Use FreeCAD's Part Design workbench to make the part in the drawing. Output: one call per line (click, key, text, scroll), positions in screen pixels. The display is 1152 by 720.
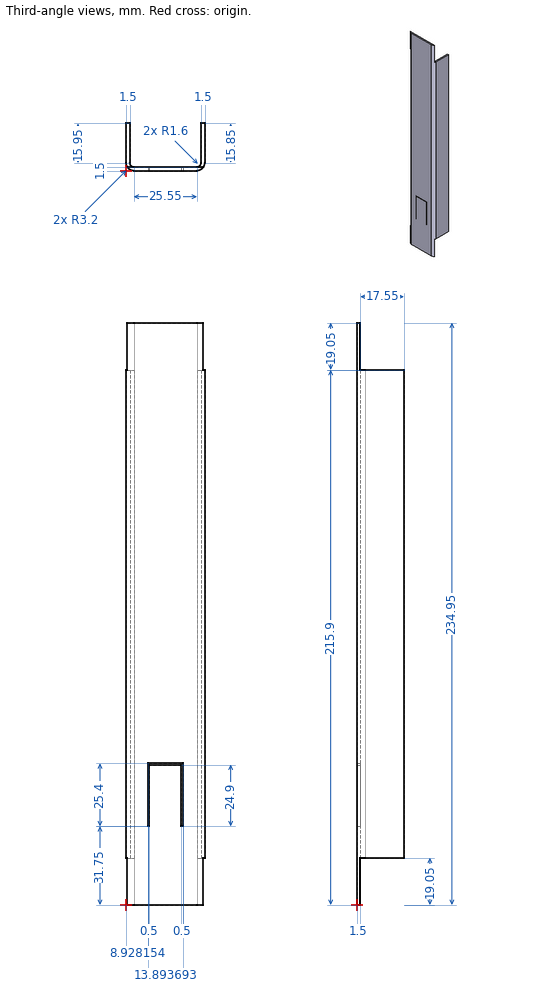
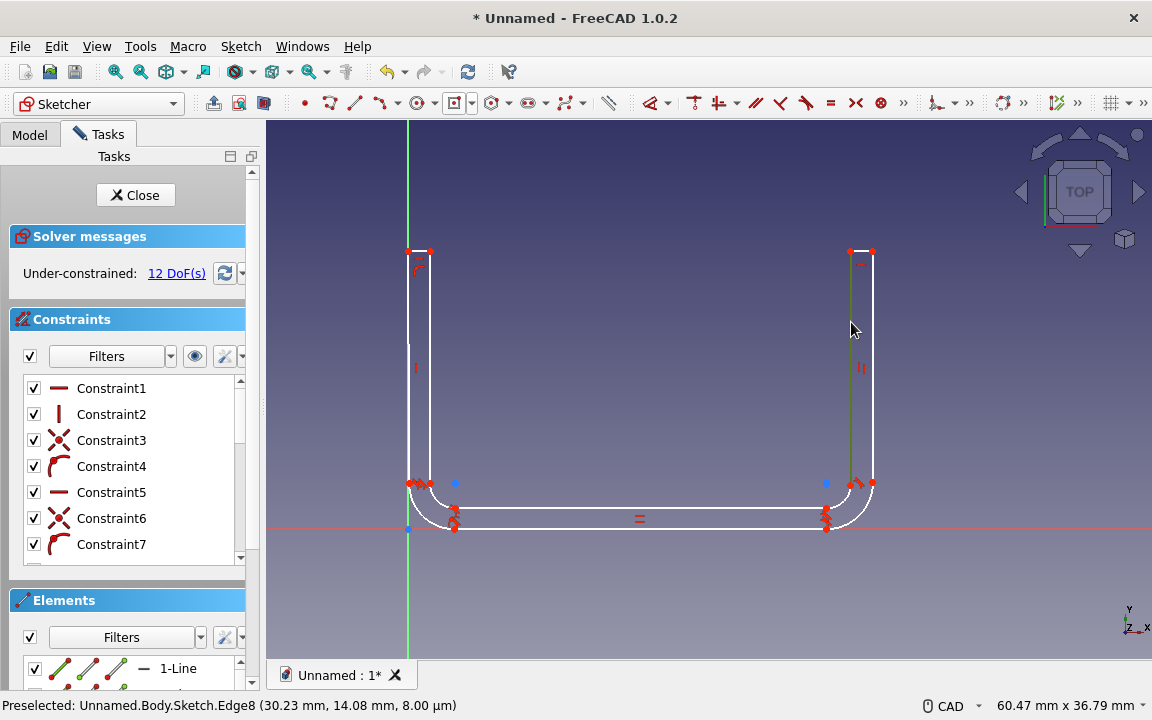
scroll(837, 506, up, 2)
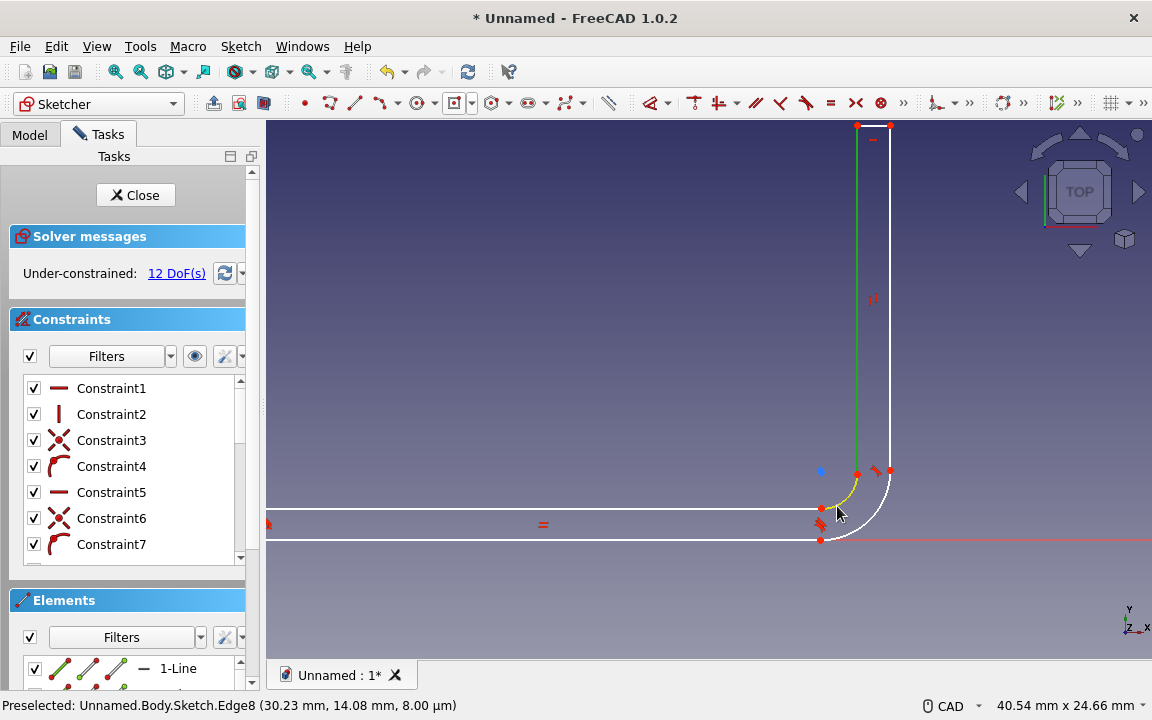
click(837, 505)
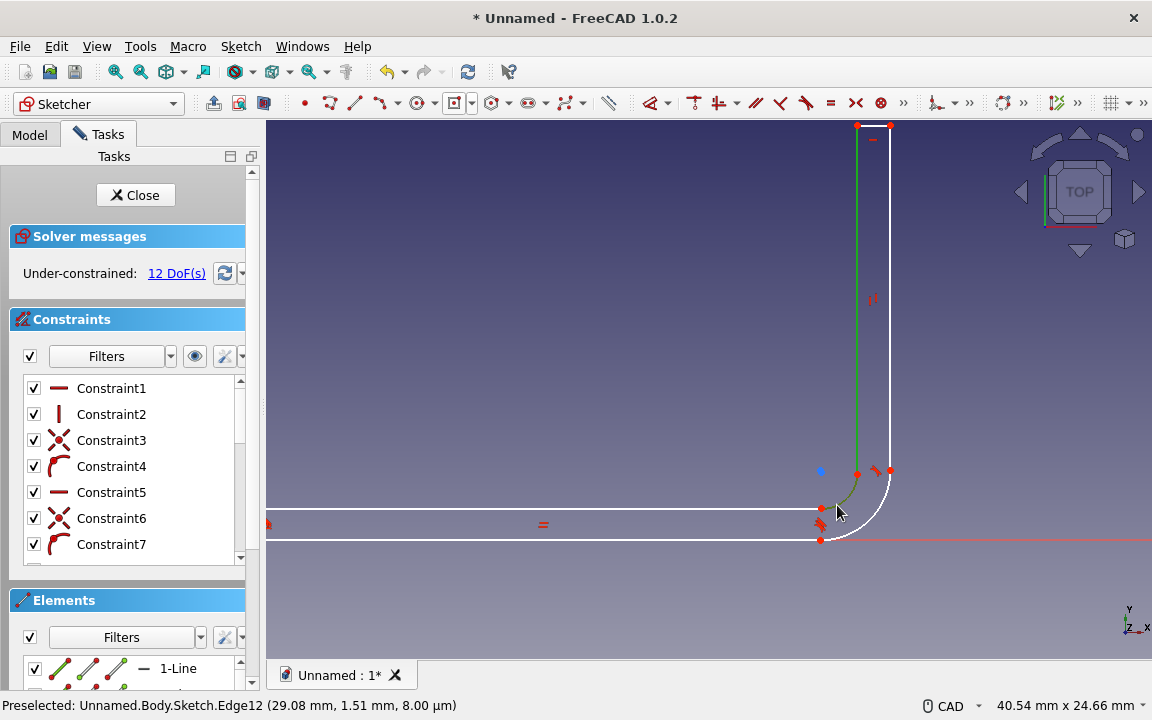
key(t)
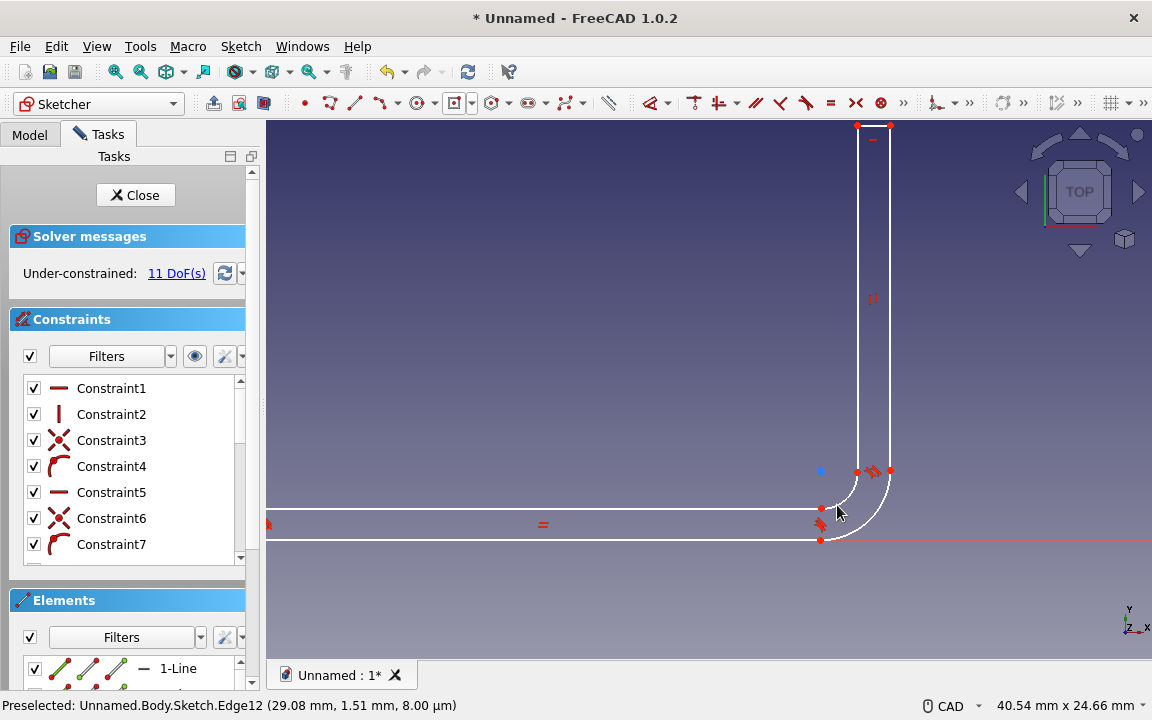
scroll(837, 506, down, 2)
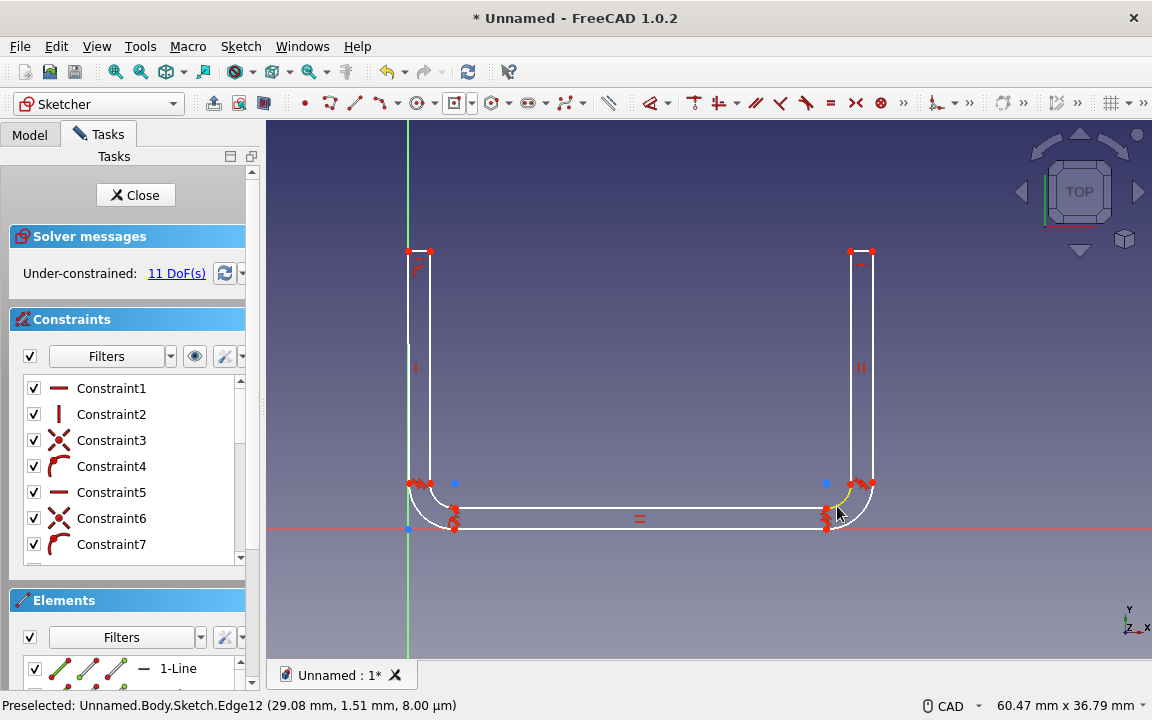
click(408, 321)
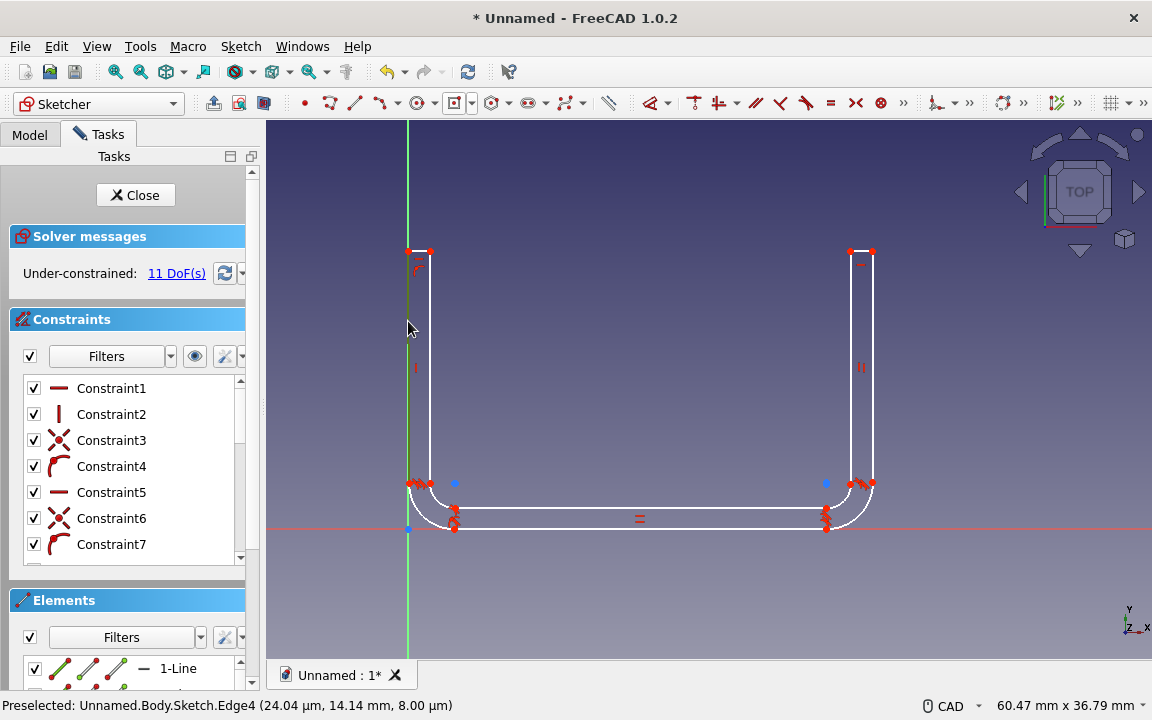
key(v)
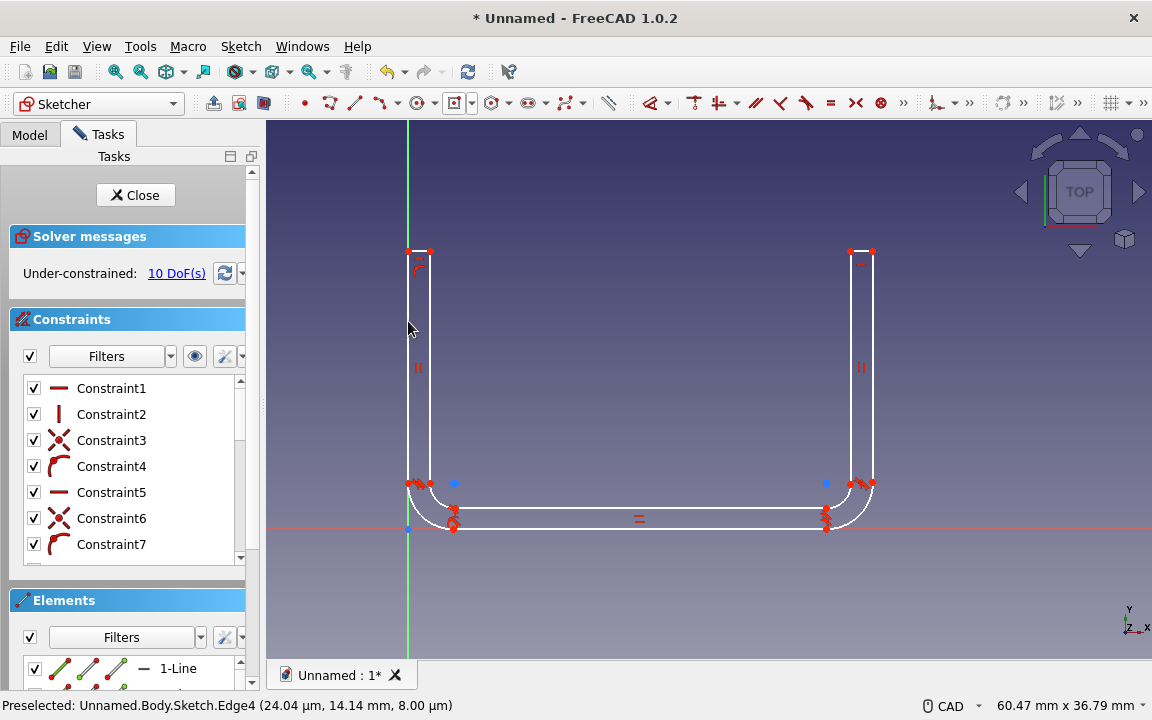
click(421, 516)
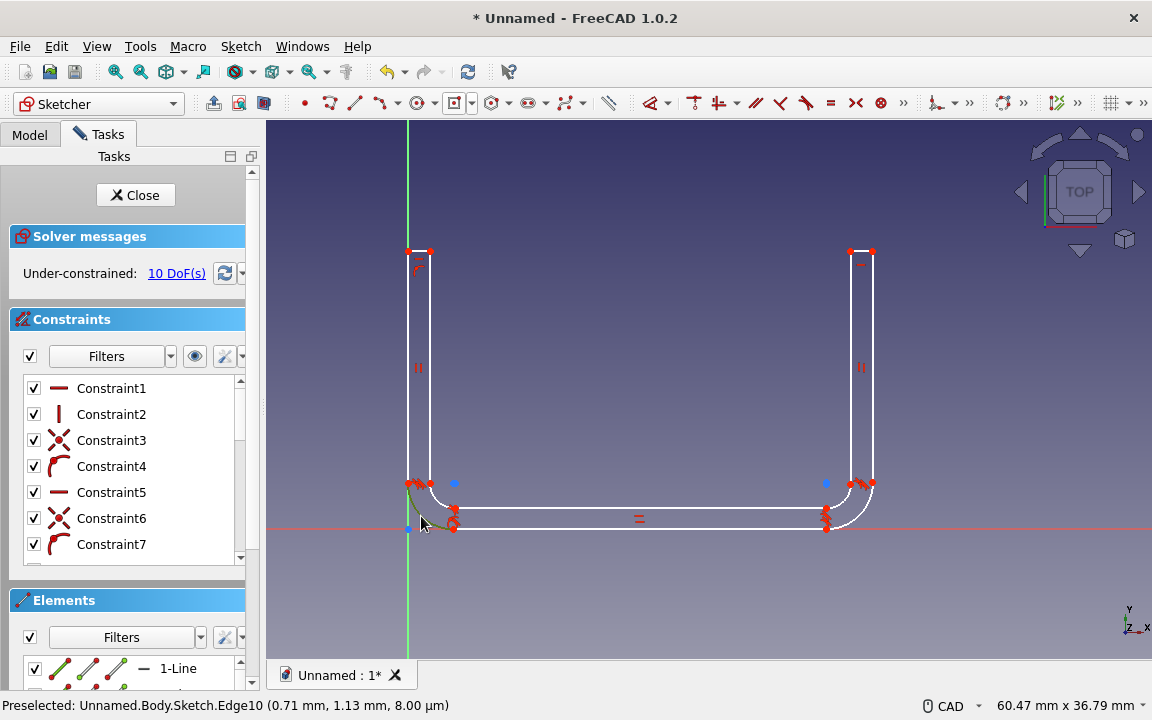
click(868, 504)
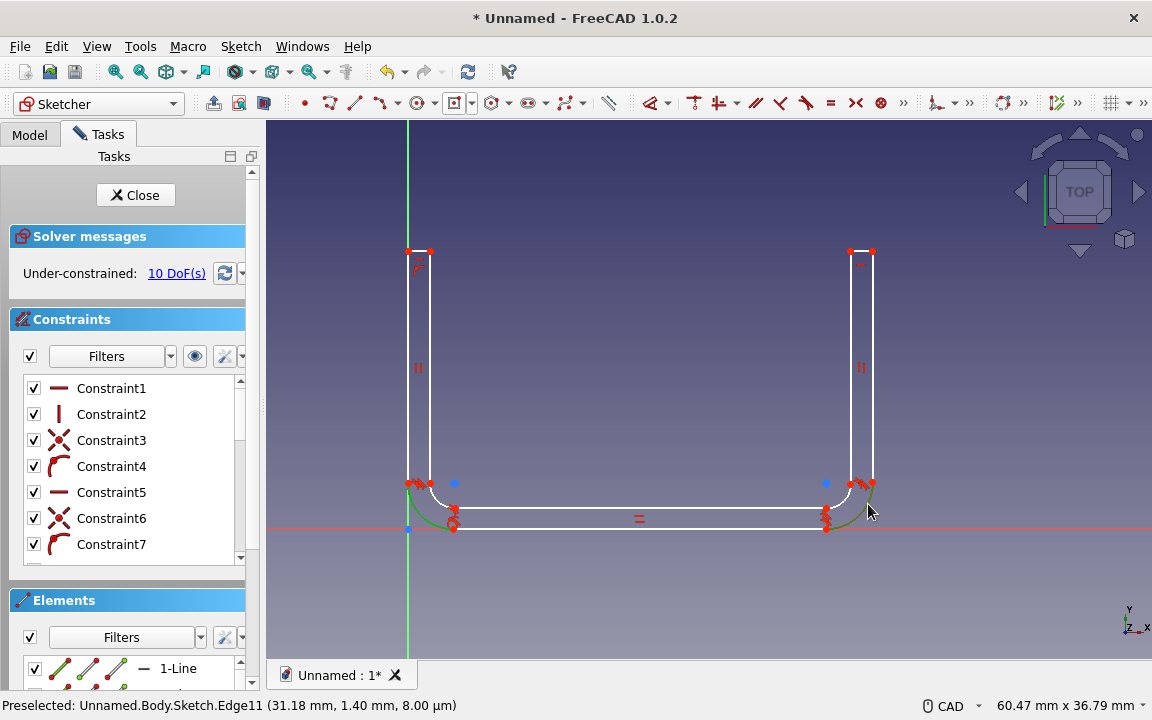
click(831, 104)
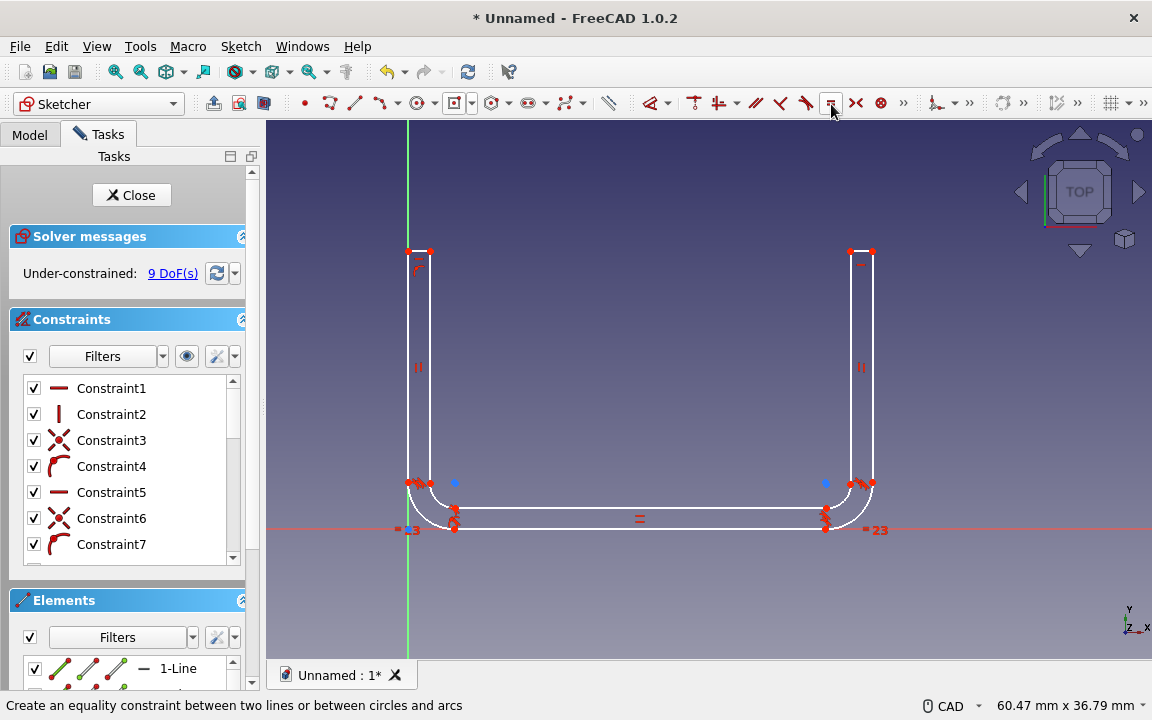
click(433, 495)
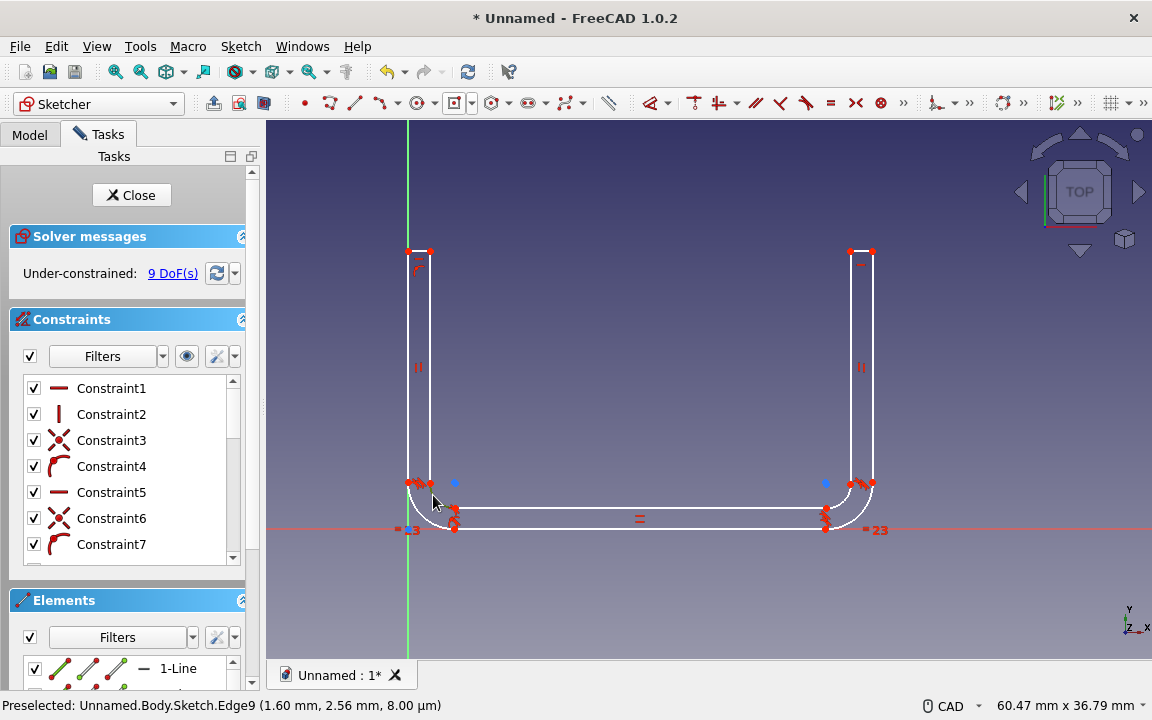
scroll(838, 506, up, 2)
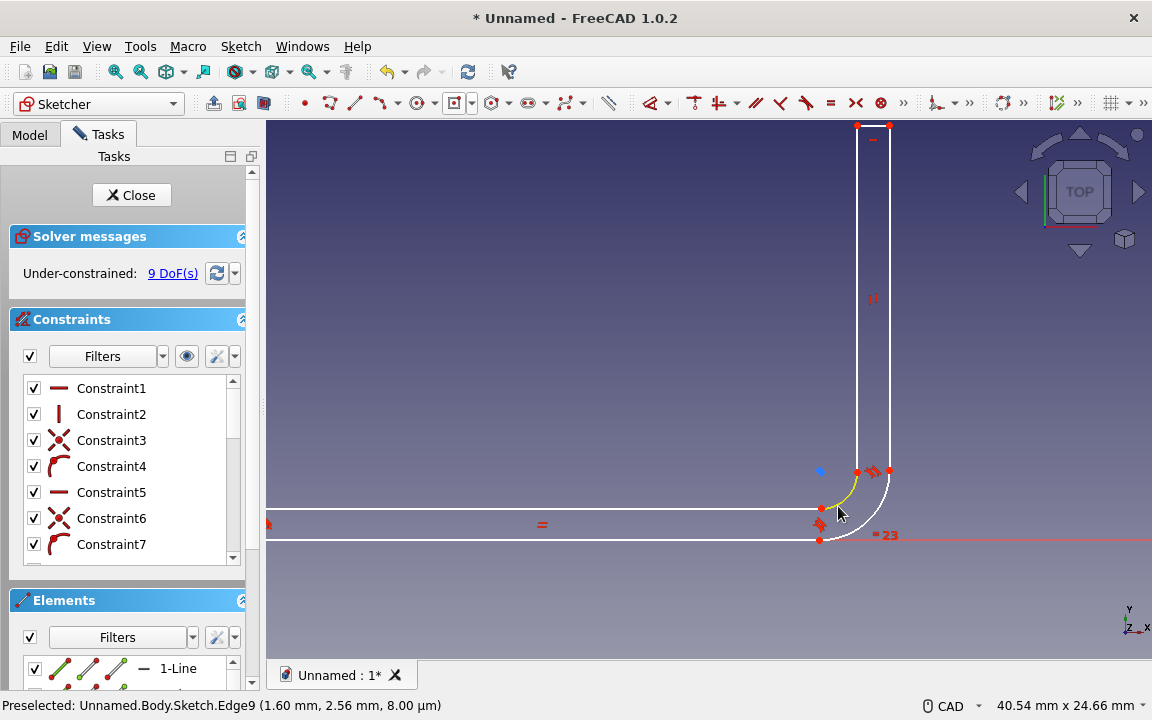
click(837, 505)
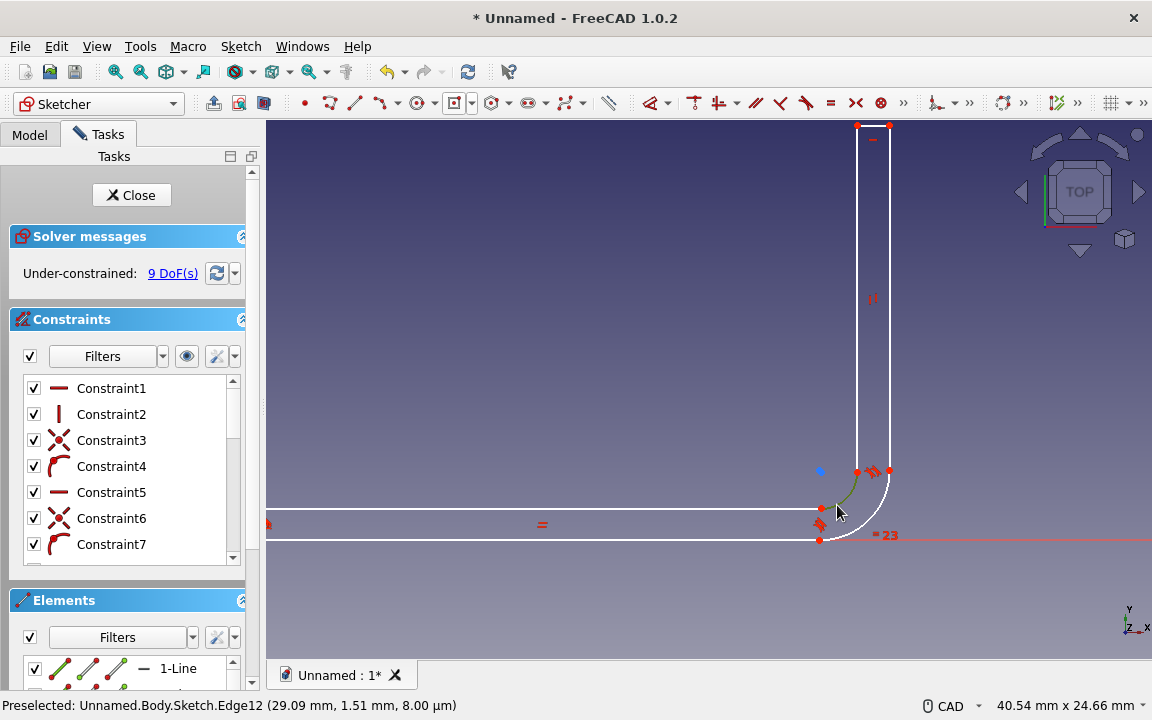
click(831, 104)